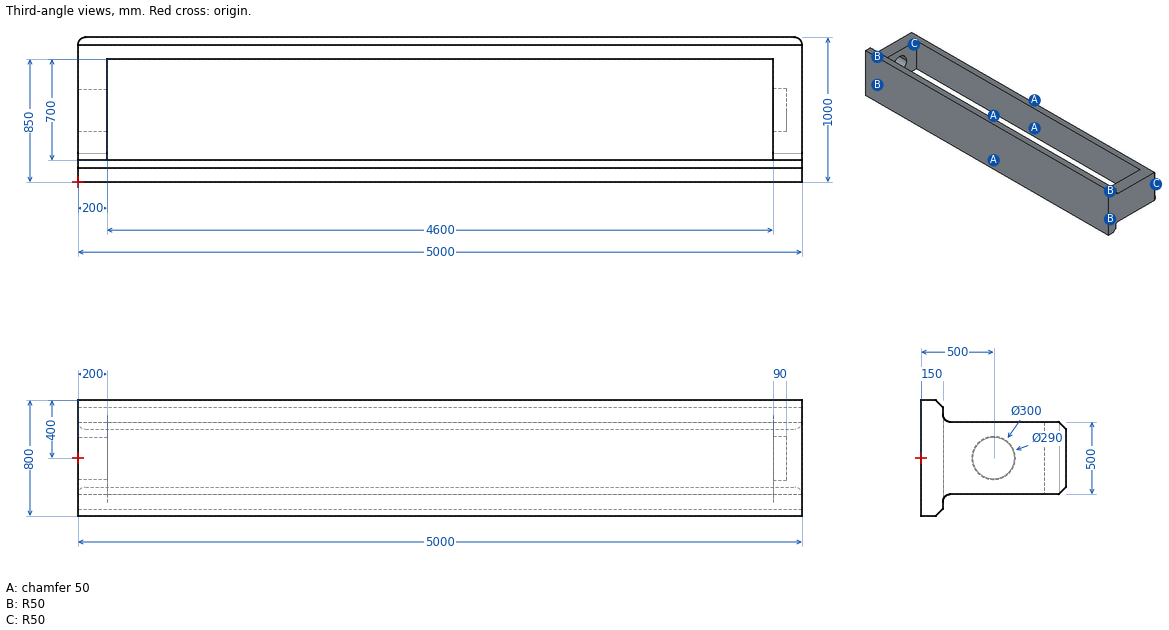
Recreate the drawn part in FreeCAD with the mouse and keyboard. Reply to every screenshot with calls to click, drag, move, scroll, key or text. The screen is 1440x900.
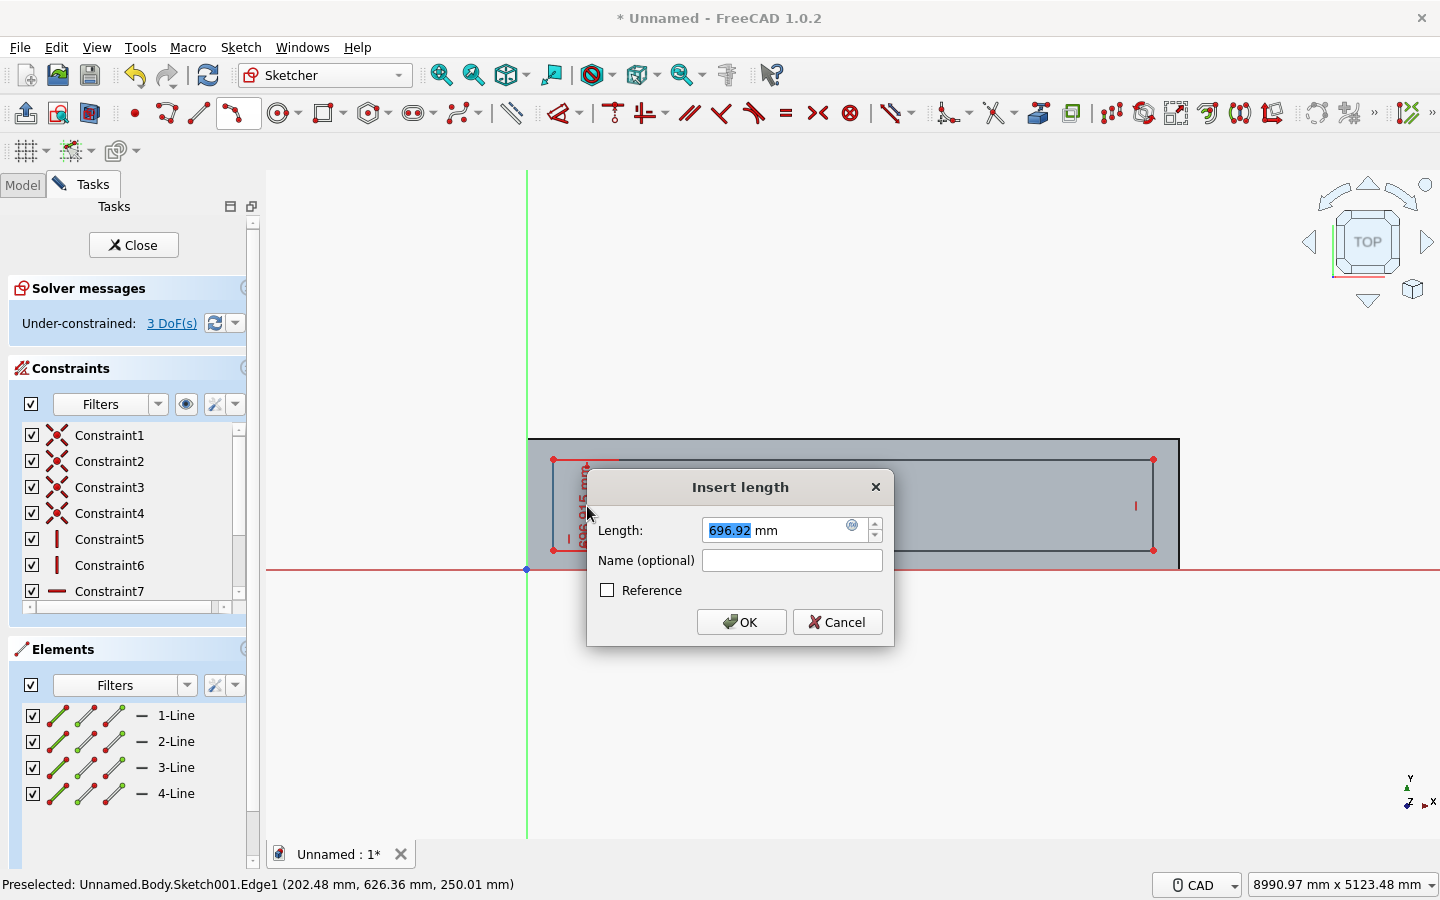
text(700)
key(Return)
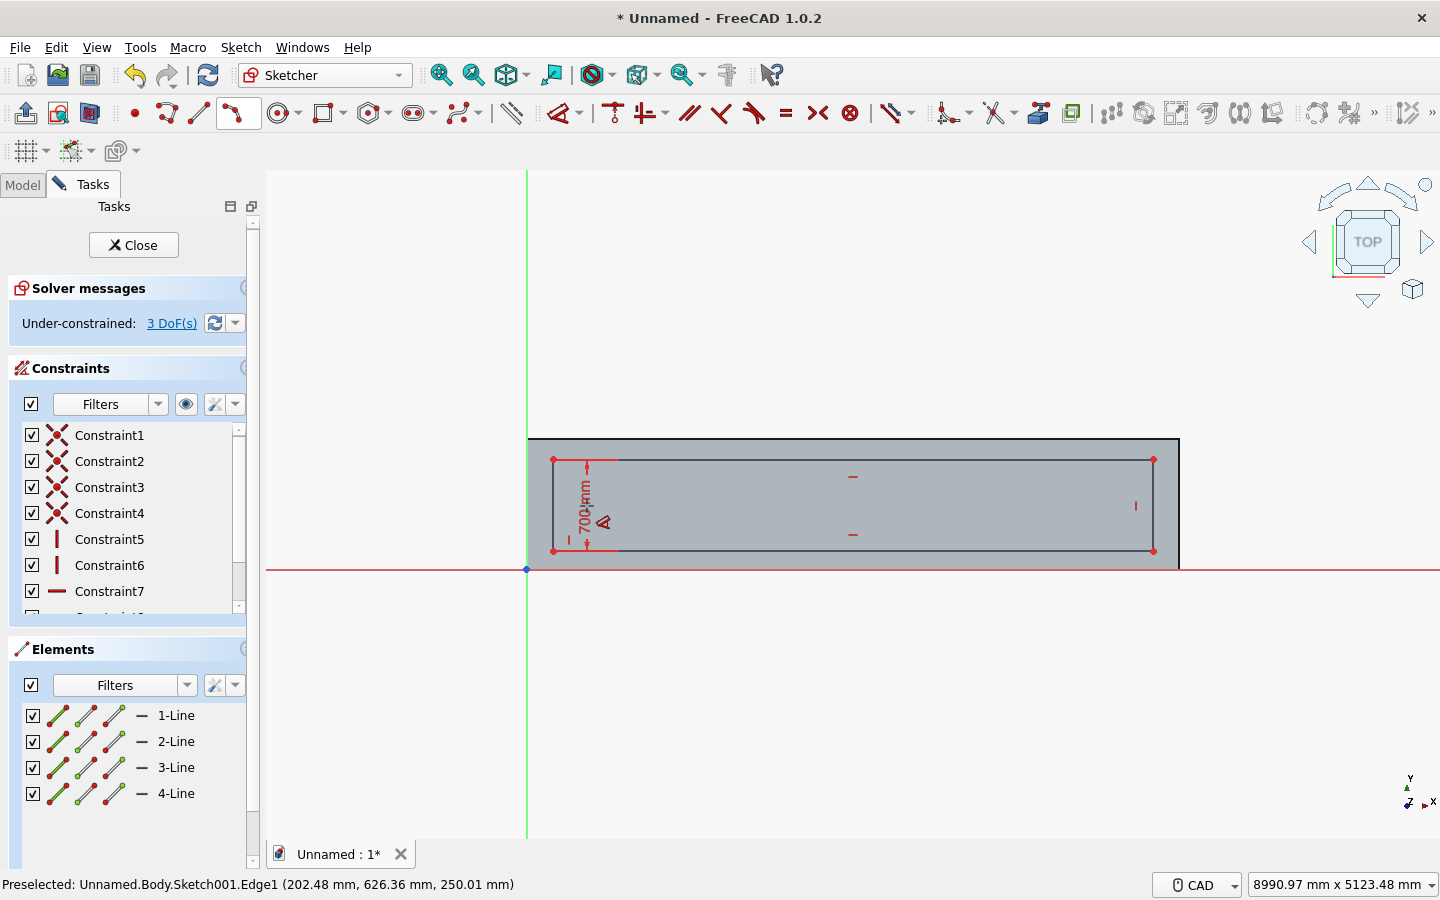
click(733, 551)
click(853, 585)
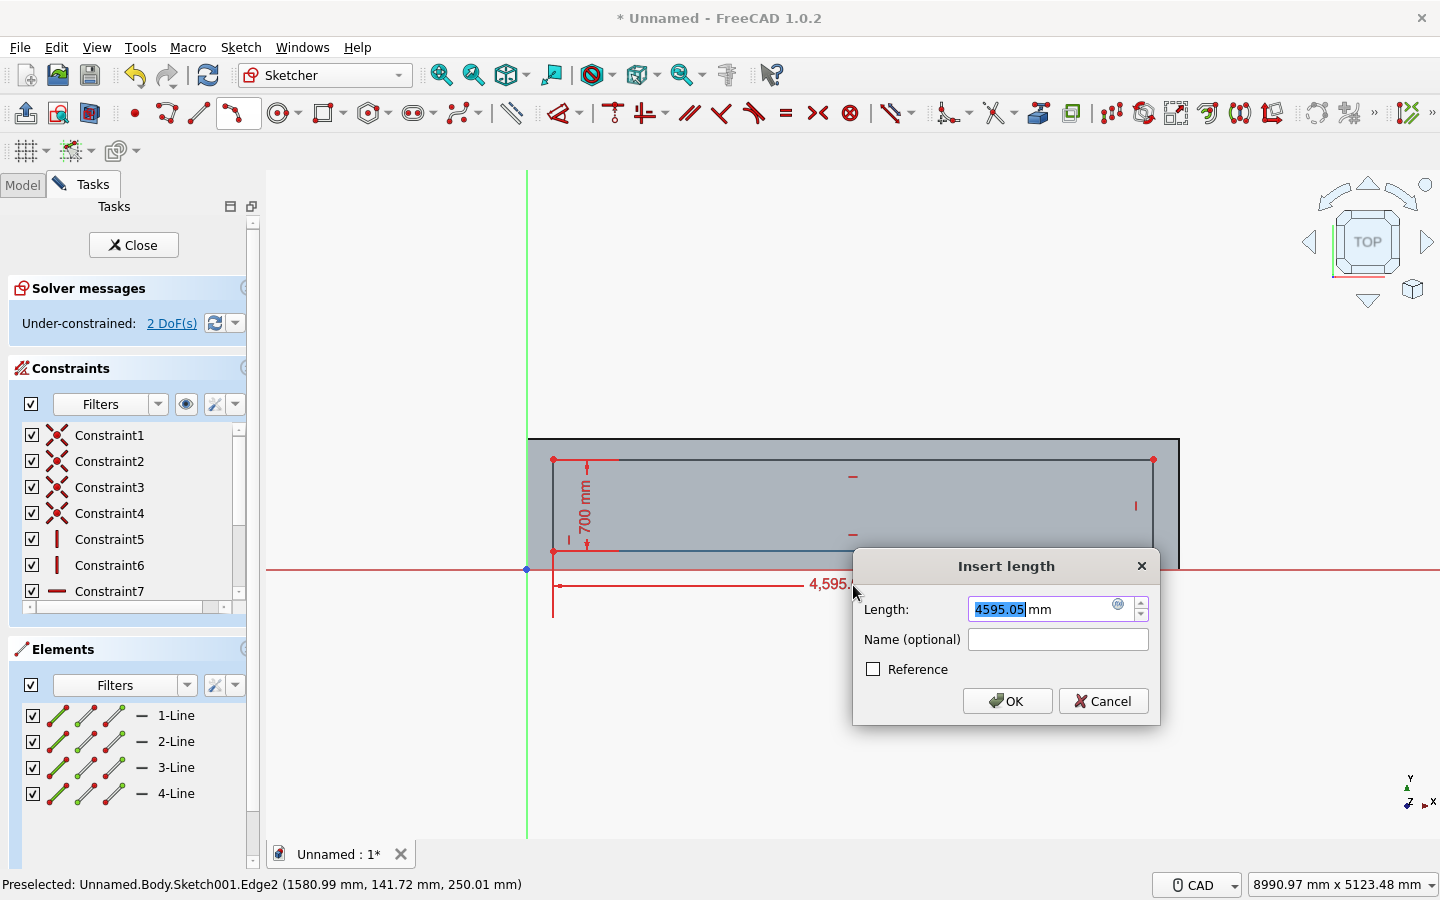
text(4600)
key(Return)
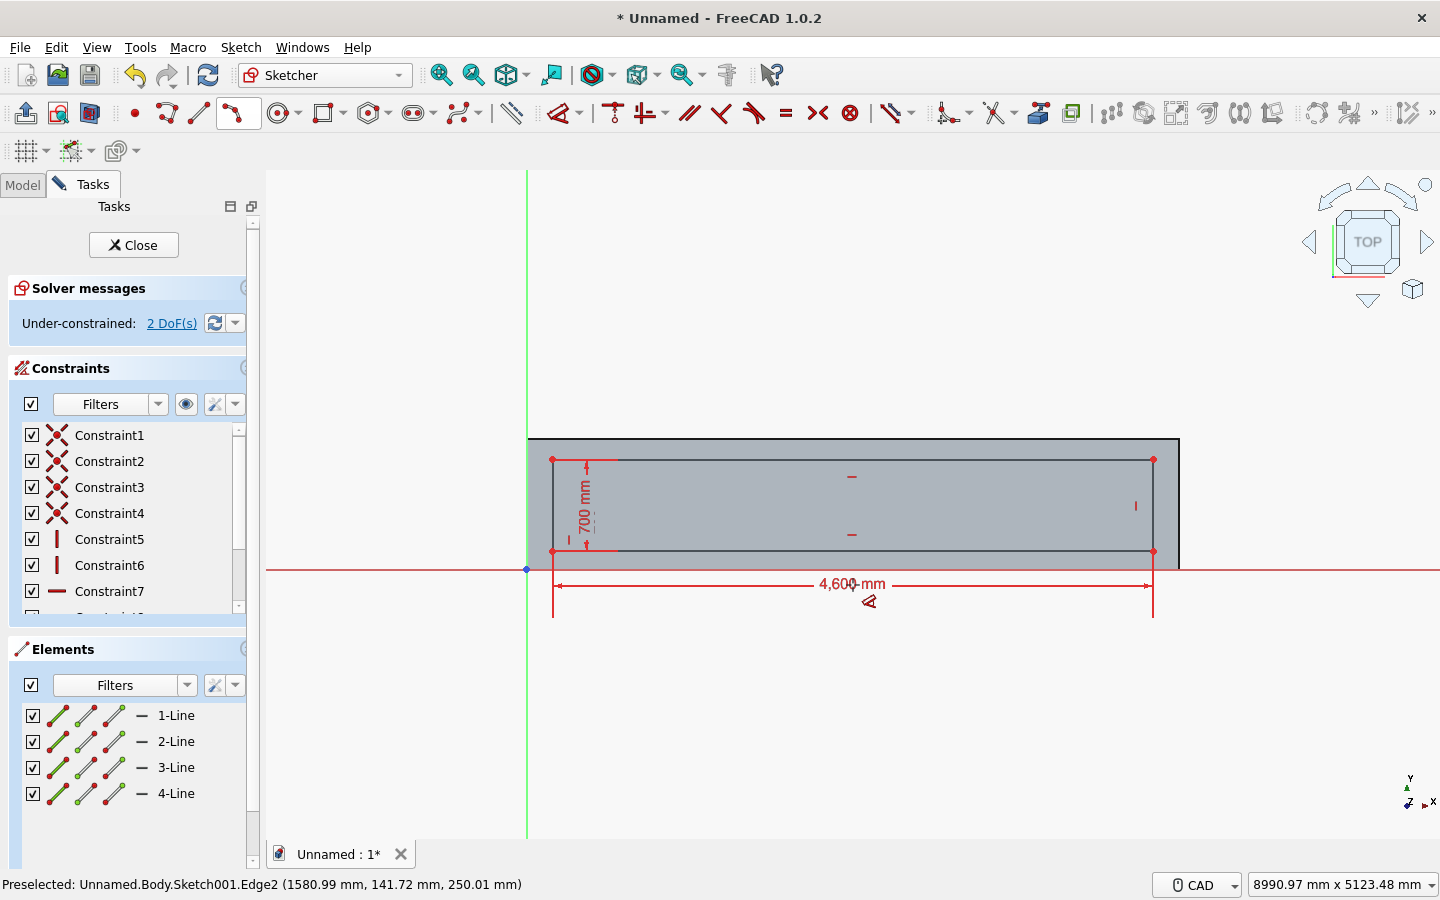
scroll(553, 460, up, 3)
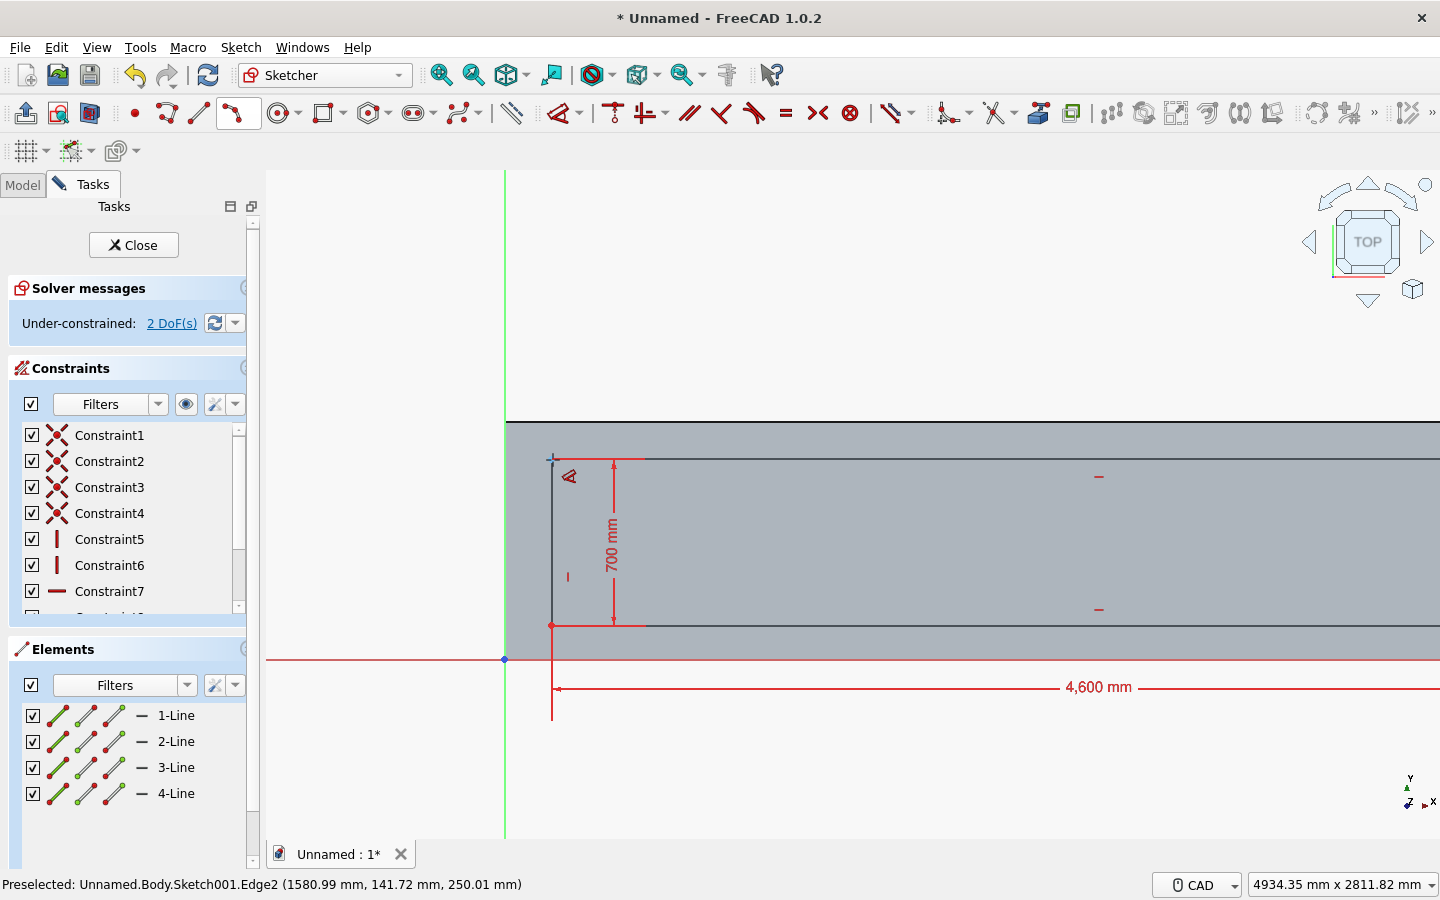
click(552, 459)
click(528, 694)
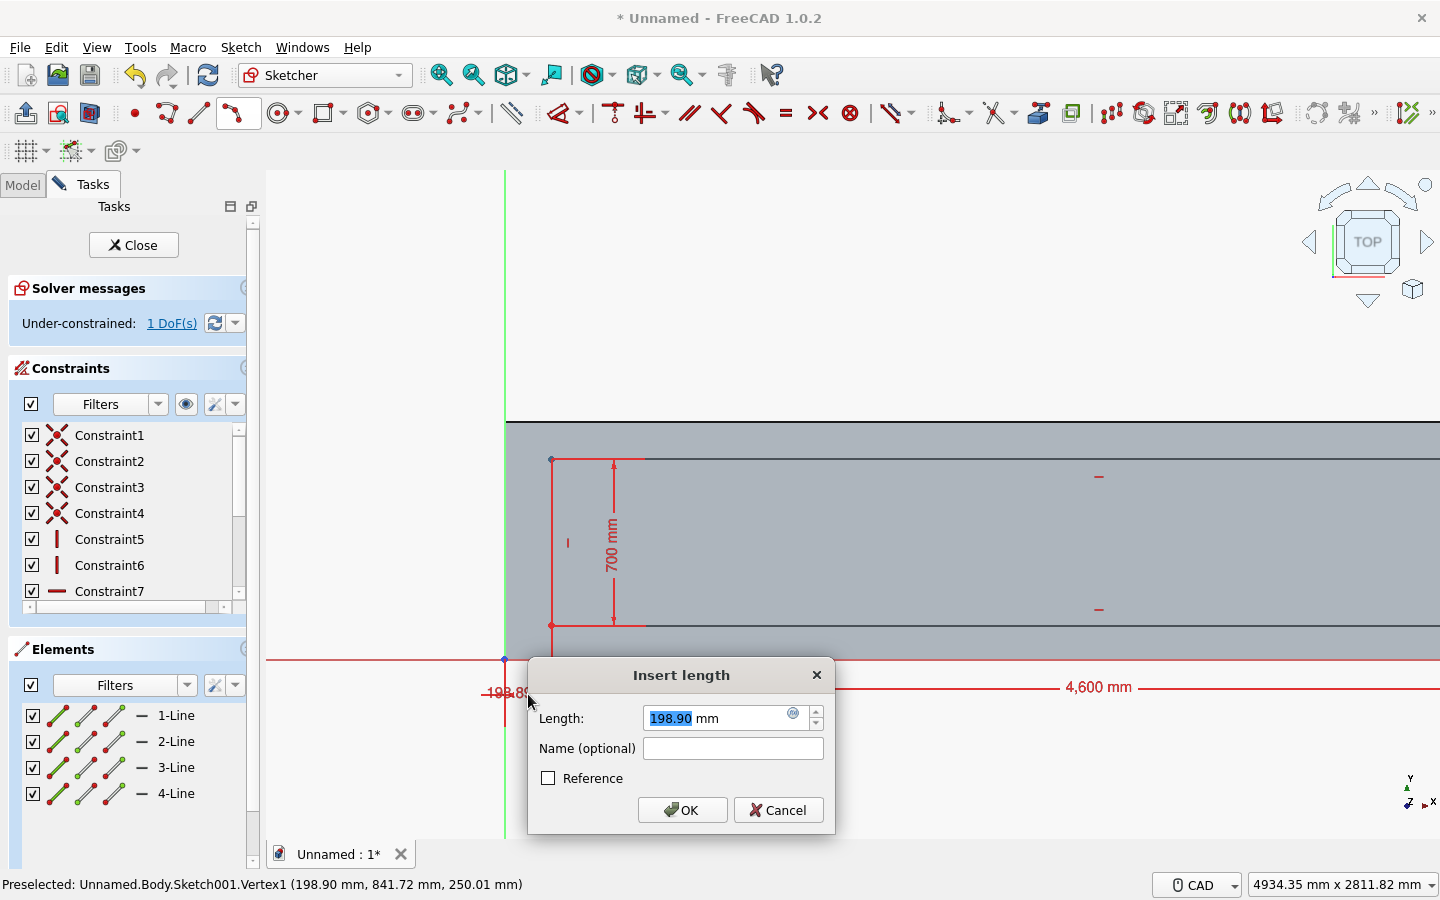
text(200)
key(Return)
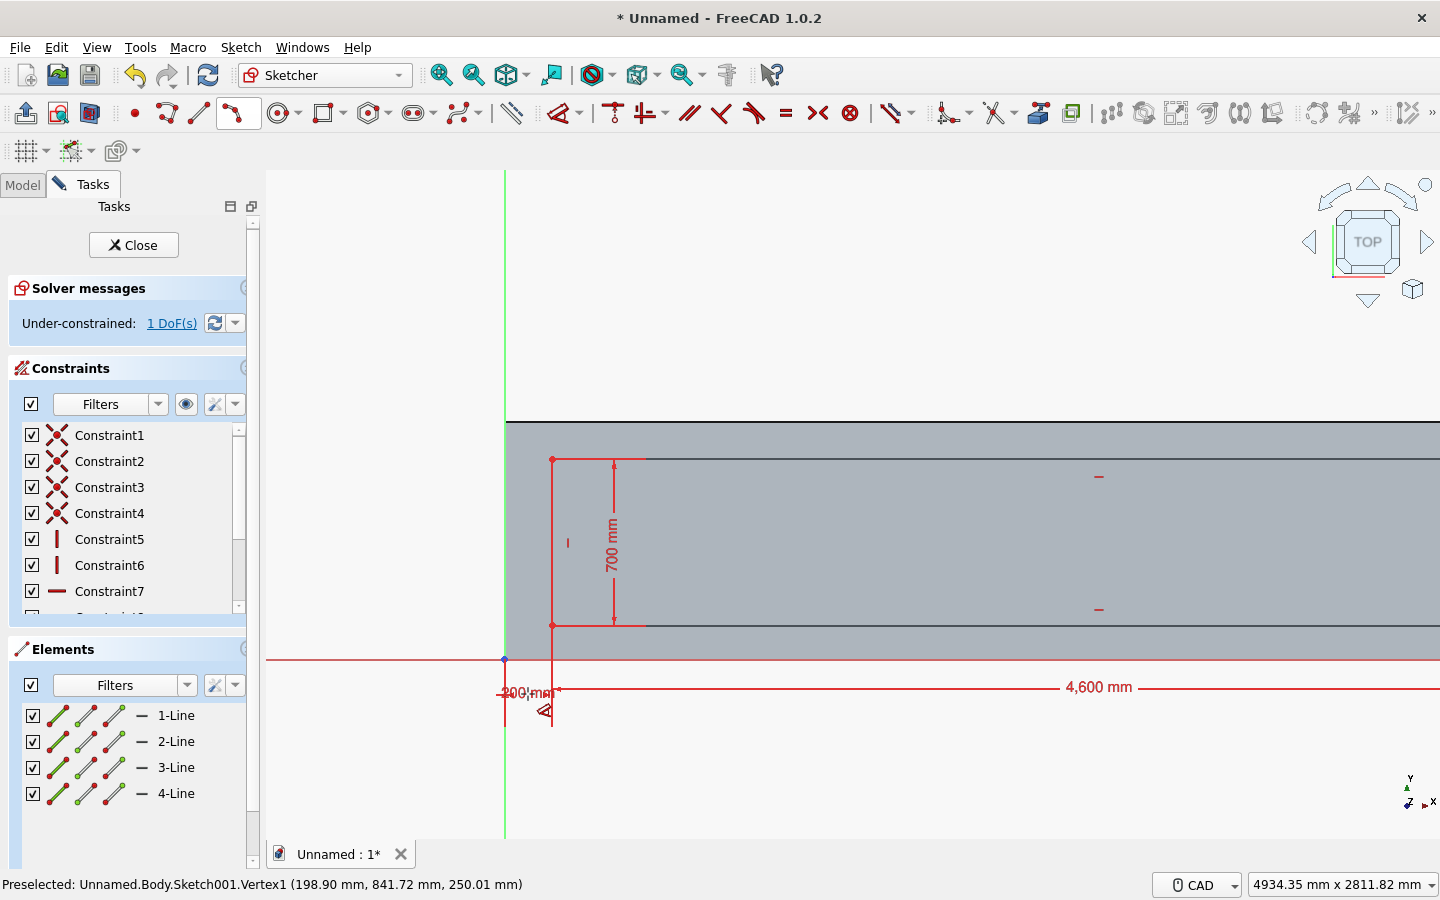
click(552, 459)
click(471, 560)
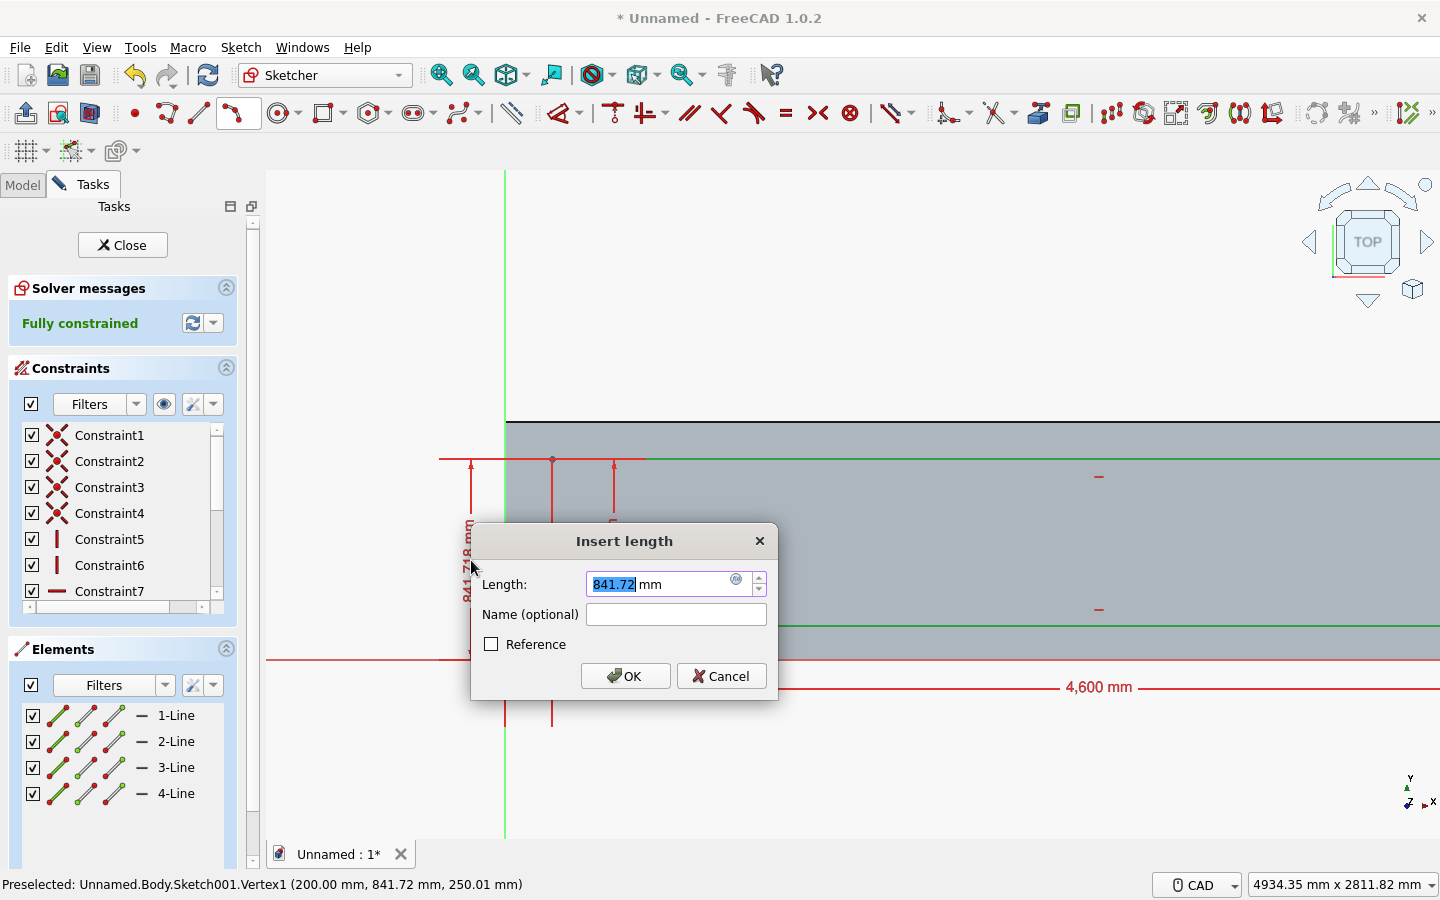
text(850)
key(Return)
key(Escape)